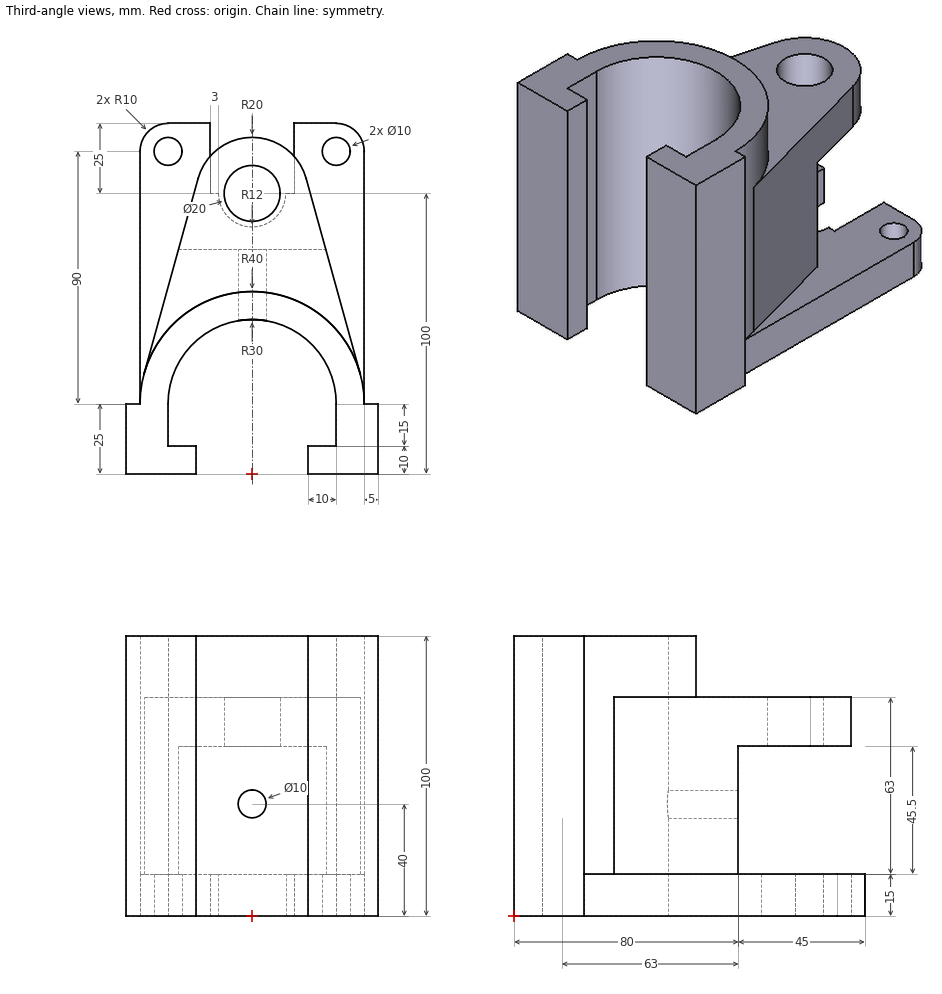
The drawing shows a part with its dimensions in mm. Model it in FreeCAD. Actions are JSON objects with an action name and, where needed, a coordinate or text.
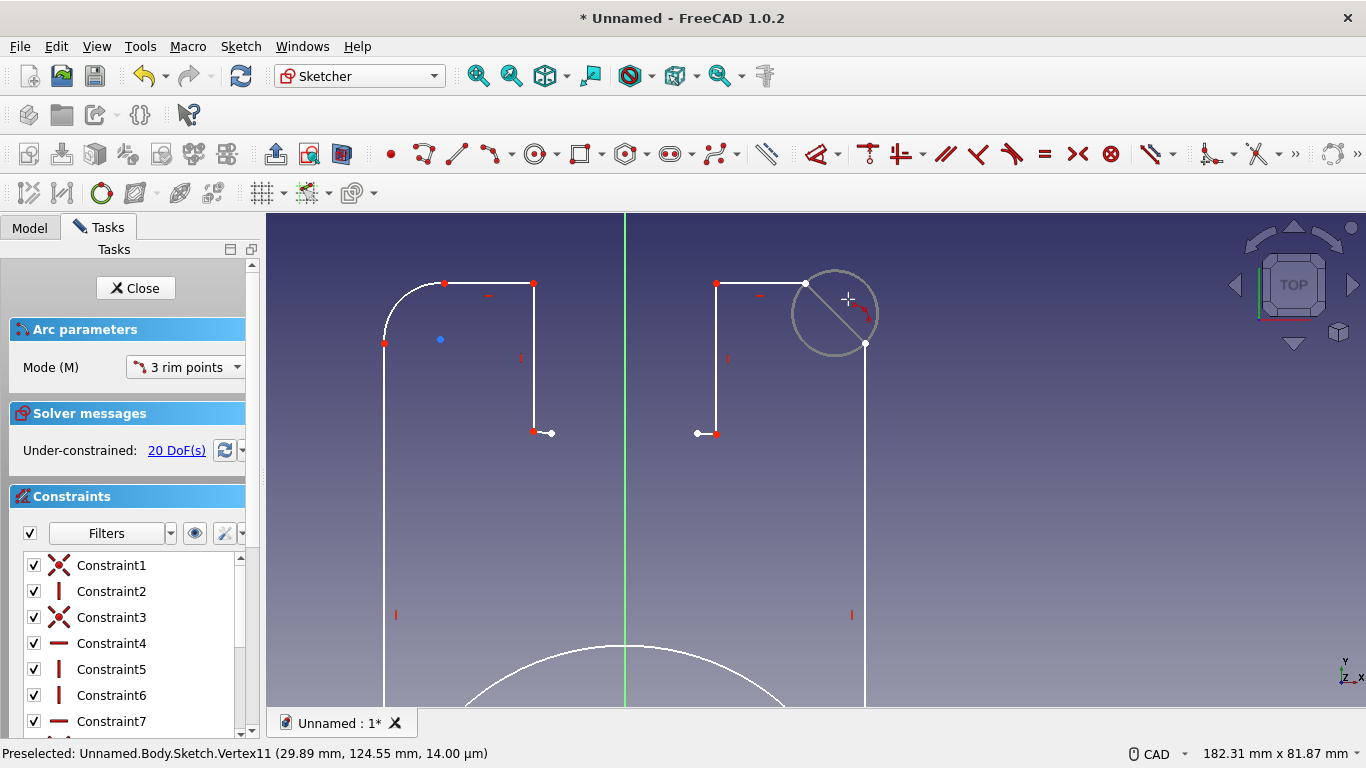
{"action": "left_click", "coordinate": [848, 298]}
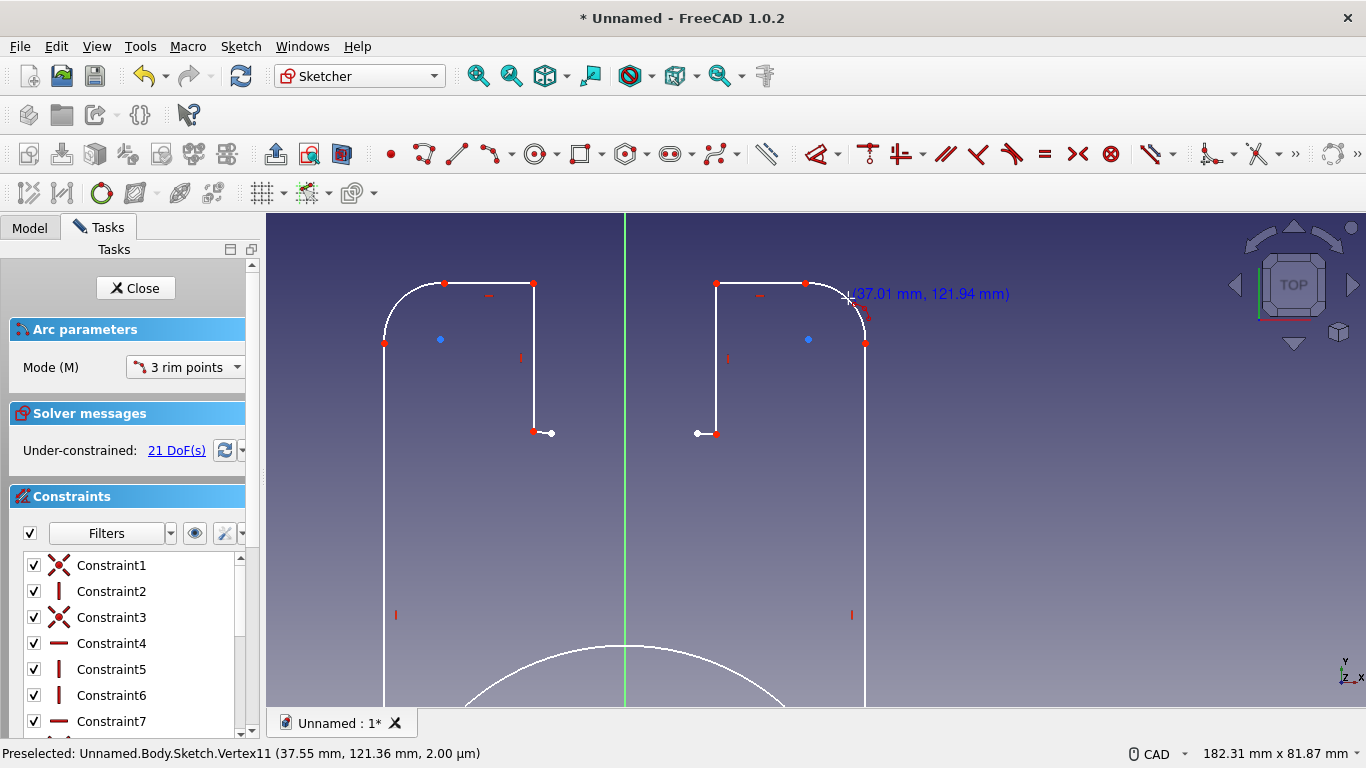
{"action": "scroll", "coordinate": [697, 431], "scroll_direction": "up", "scroll_amount": 3}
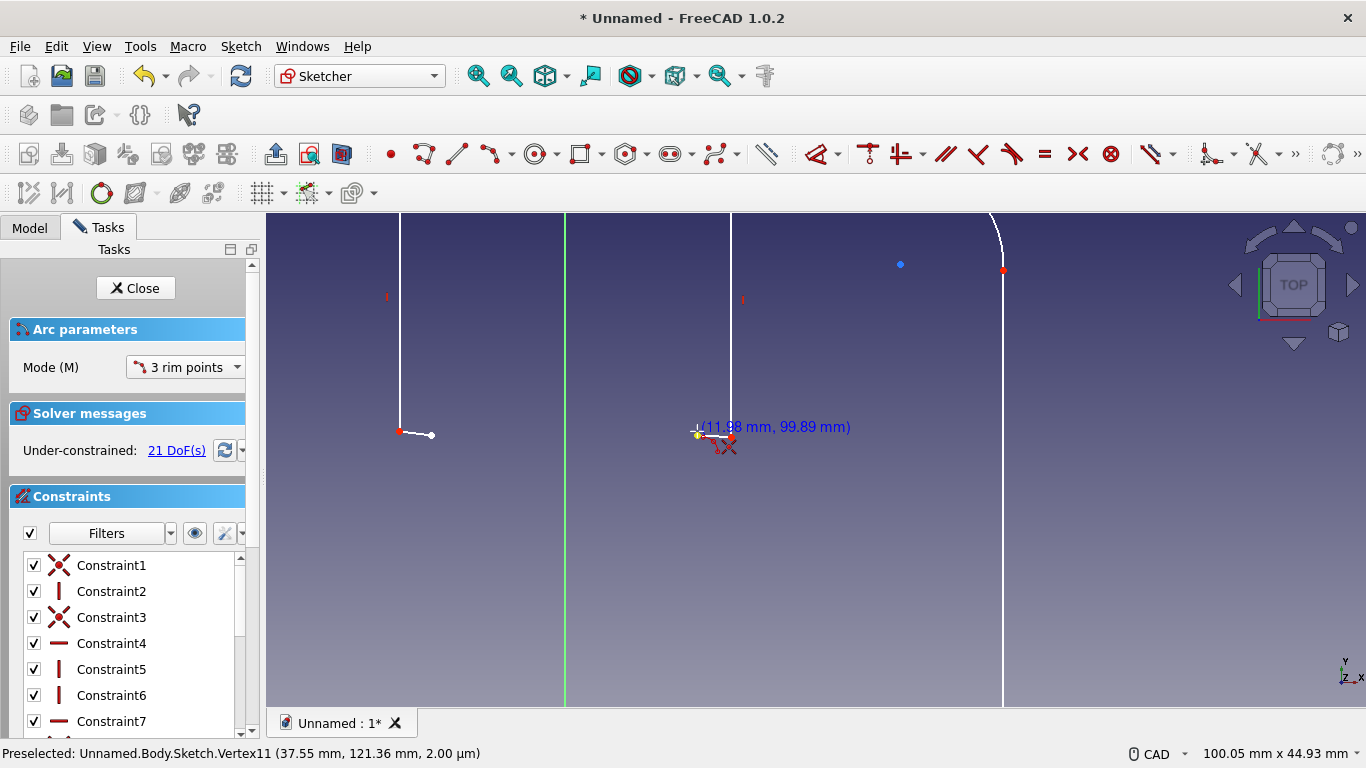
{"action": "left_click", "coordinate": [698, 436]}
{"action": "left_click", "coordinate": [432, 435]}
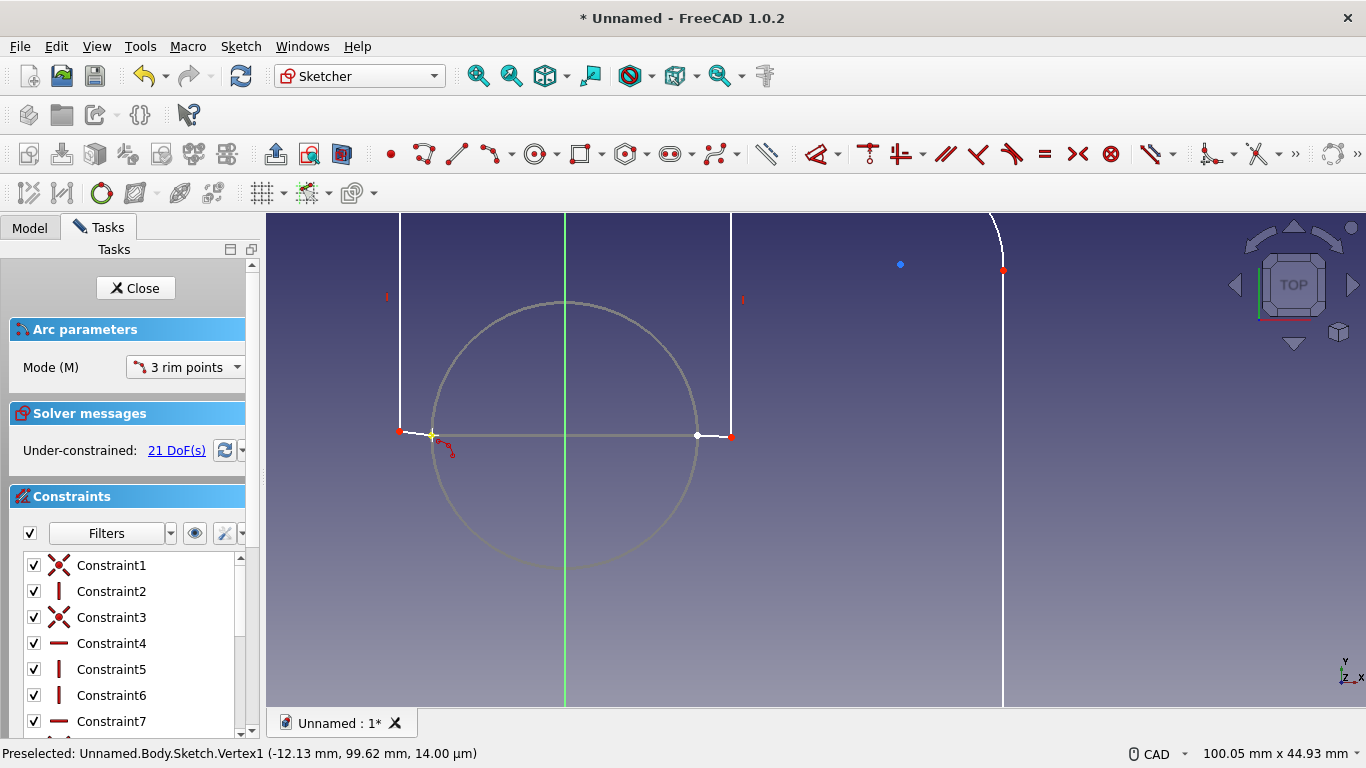
{"action": "scroll", "coordinate": [807, 334], "scroll_direction": "down", "scroll_amount": 7}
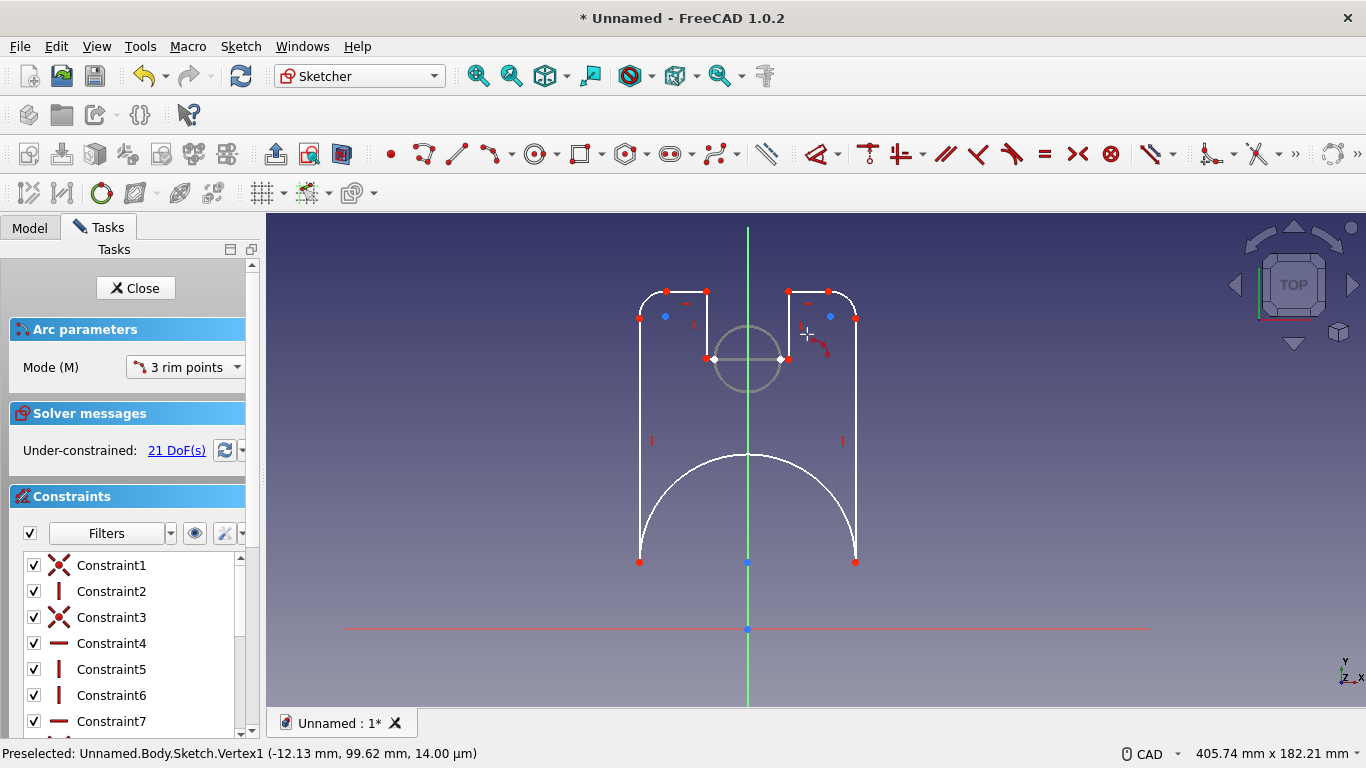
{"action": "left_click", "coordinate": [729, 384]}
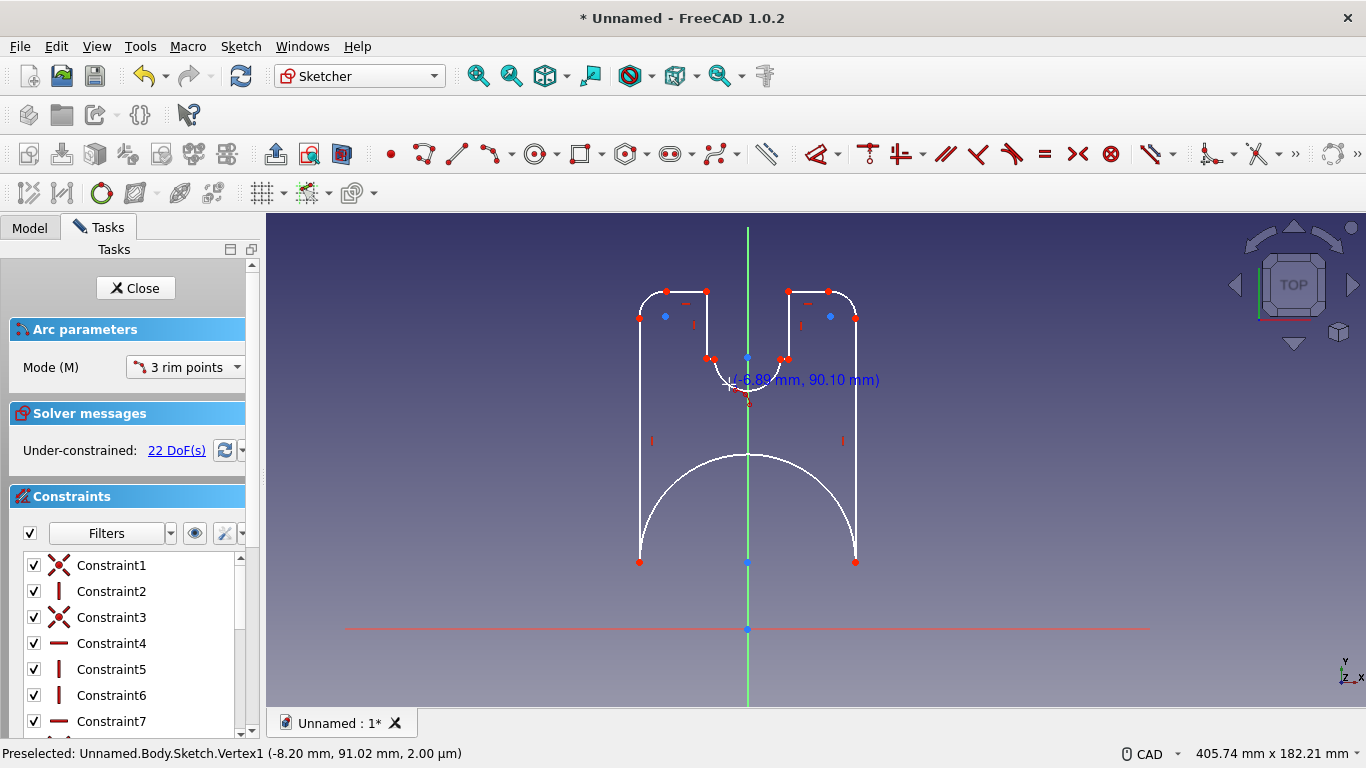
{"action": "key", "text": "g c"}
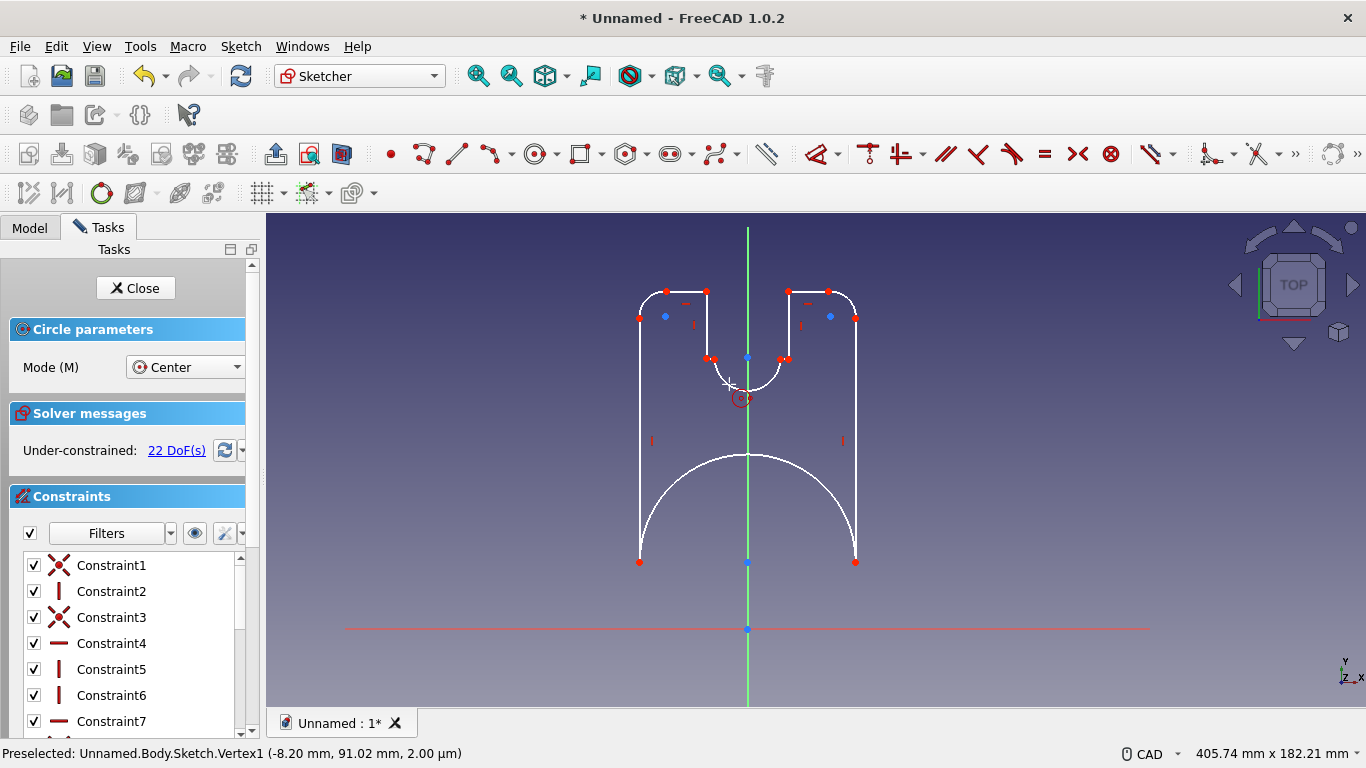
{"action": "scroll", "coordinate": [829, 318], "scroll_direction": "up", "scroll_amount": 3}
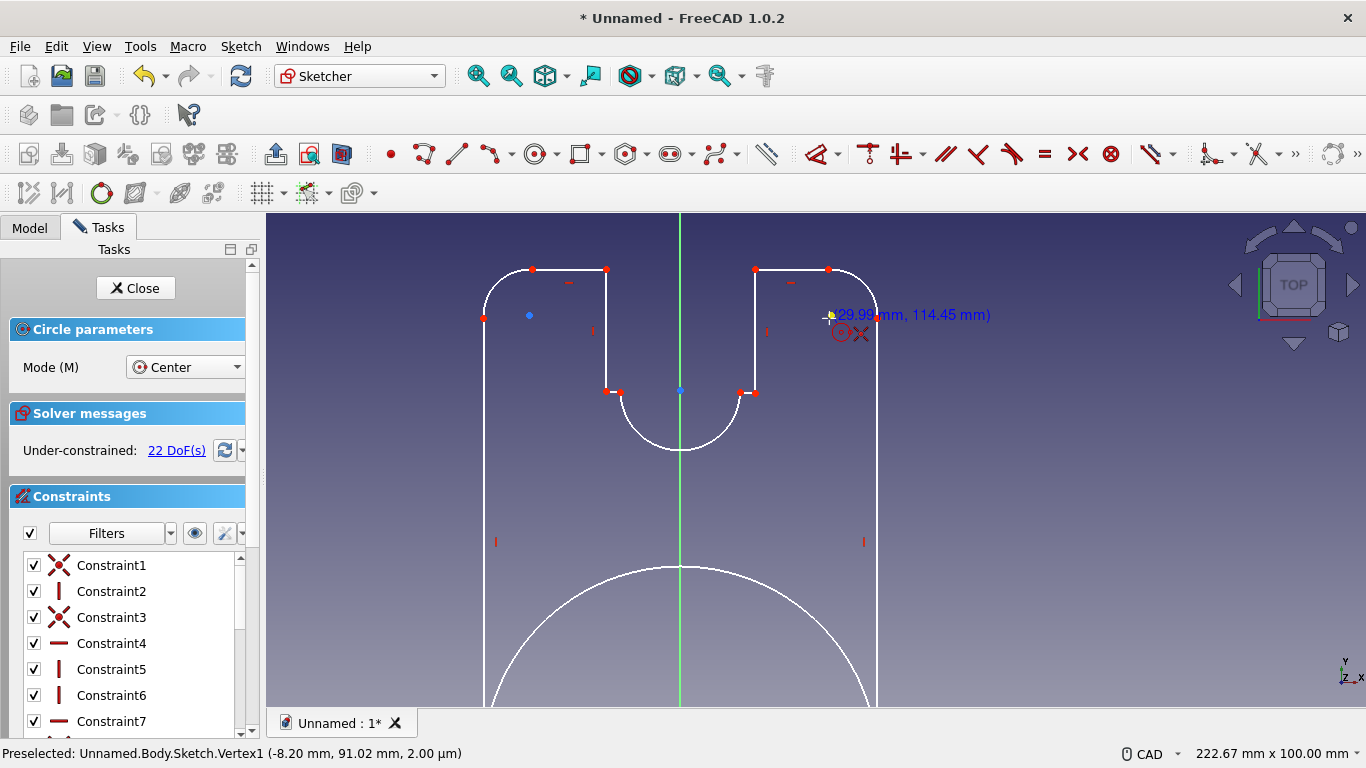
{"action": "left_click", "coordinate": [829, 317]}
{"action": "mouse_move", "coordinate": [846, 299]}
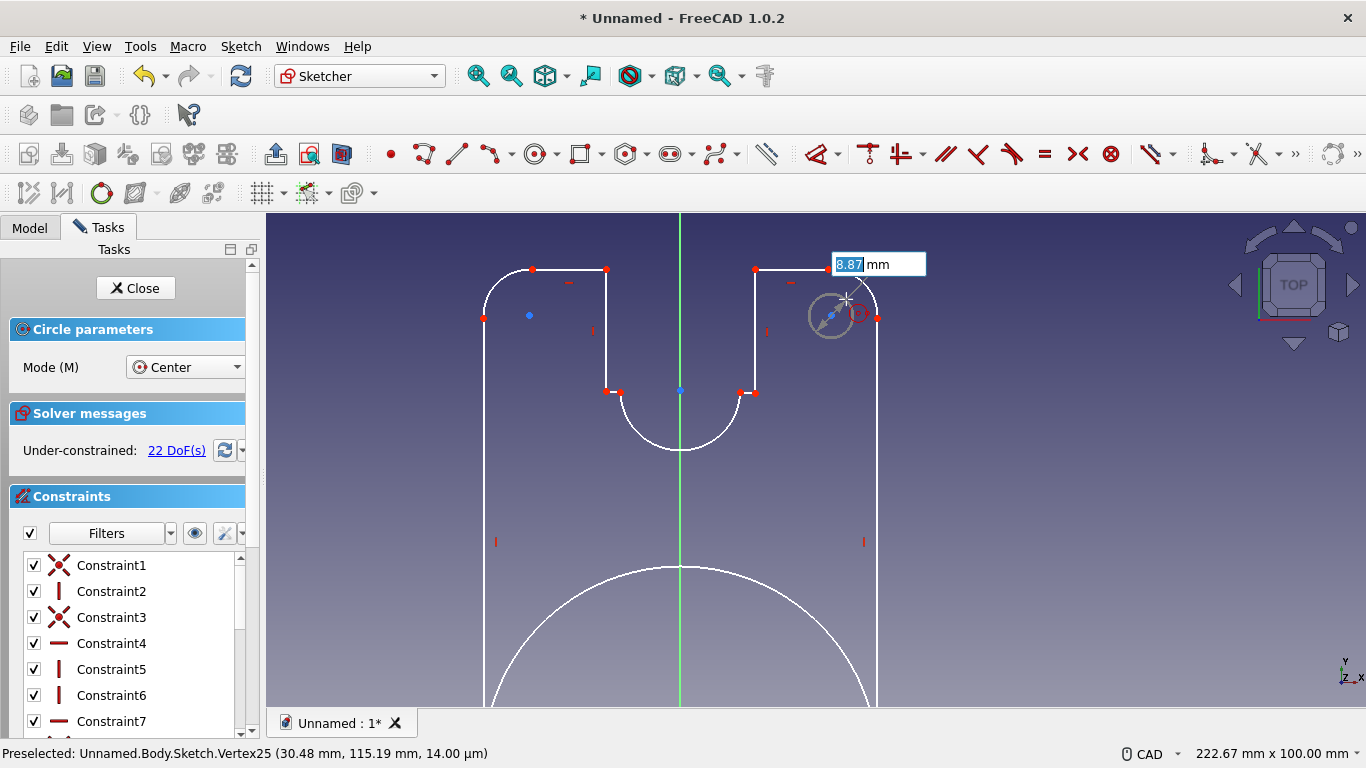
{"action": "type", "text": "10"}
{"action": "key", "text": "Return"}